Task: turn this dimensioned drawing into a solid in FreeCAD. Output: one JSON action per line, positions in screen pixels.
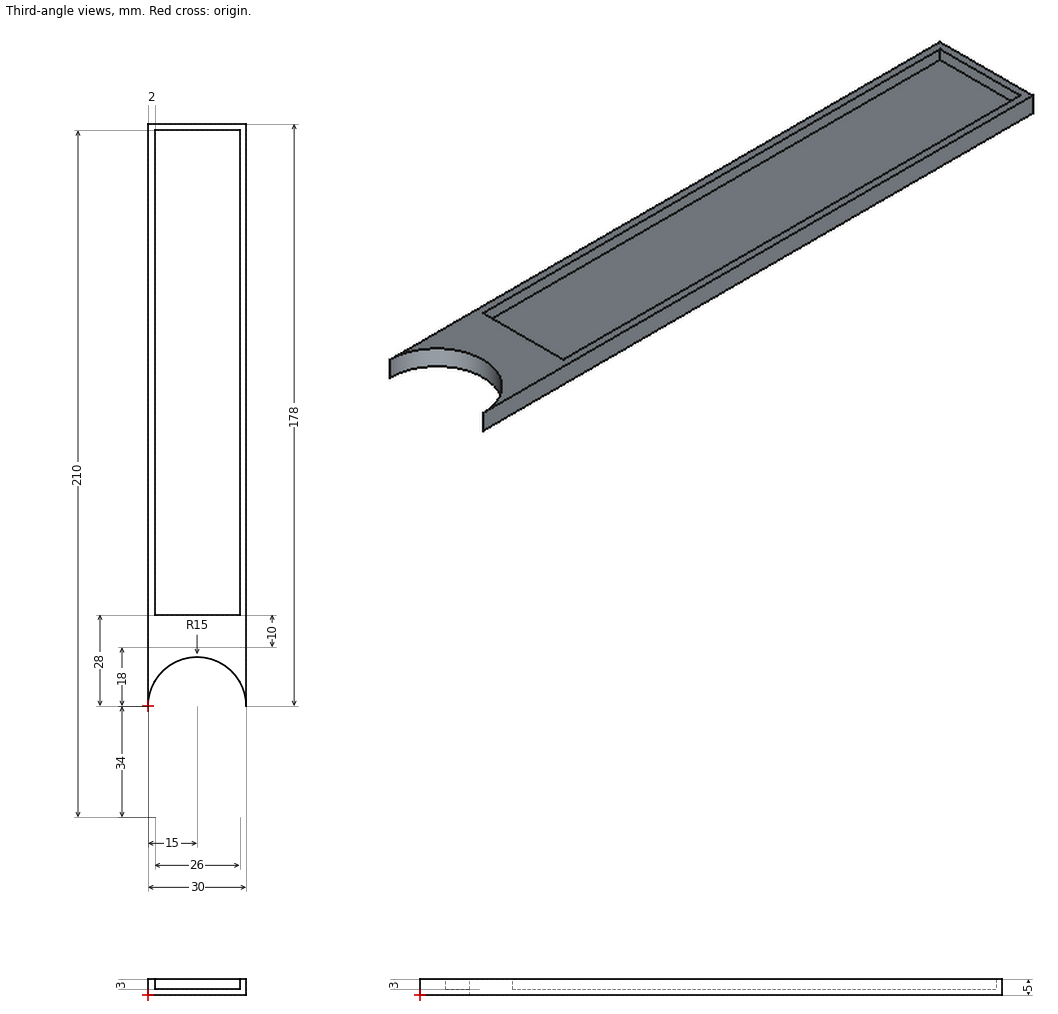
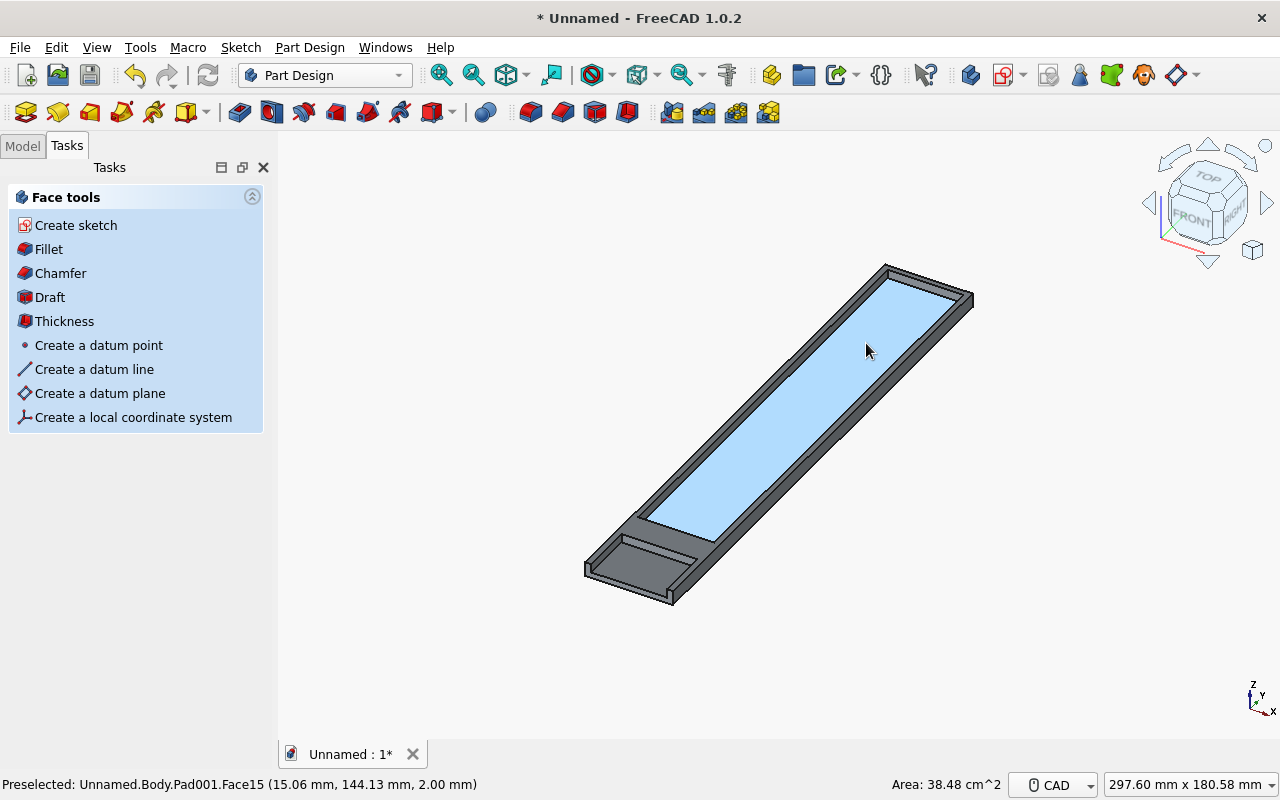
{"action": "left_click", "coordinate": [1004, 76]}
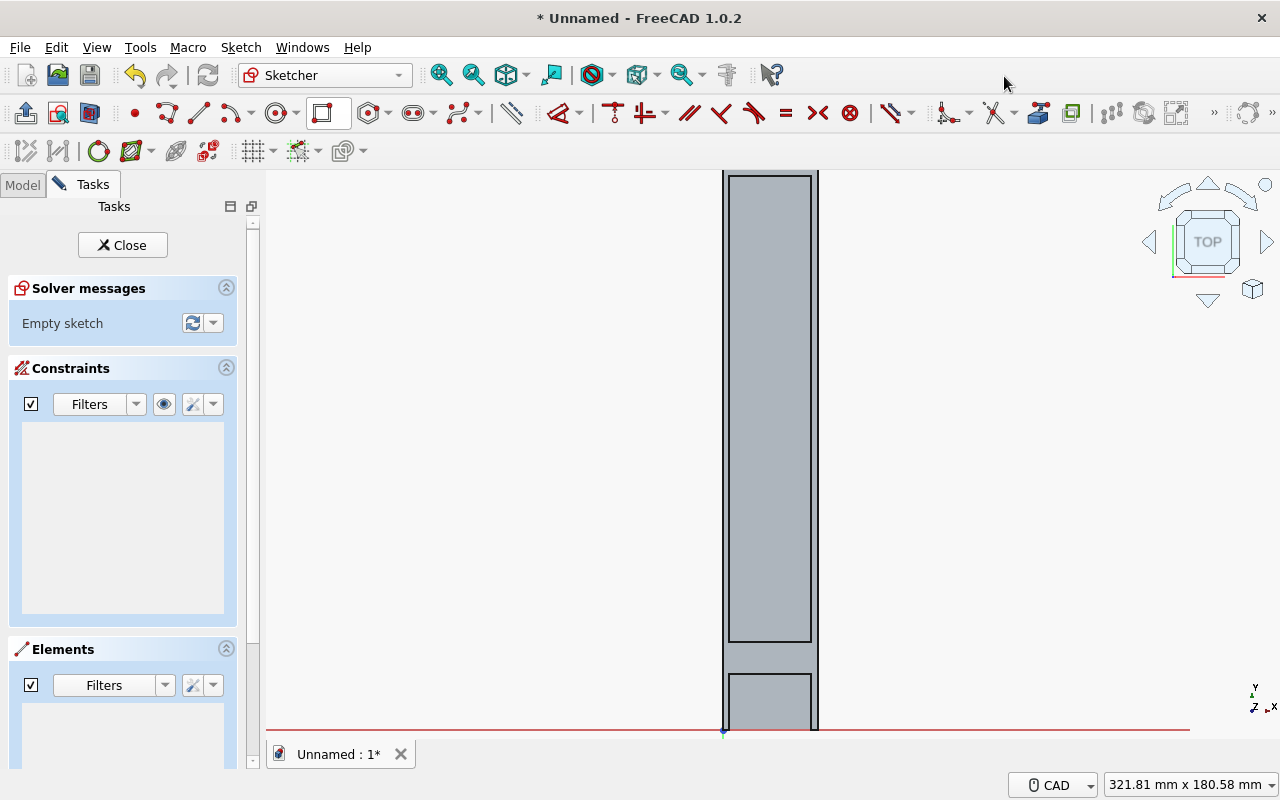
{"action": "scroll", "coordinate": [704, 454], "scroll_direction": "down", "scroll_amount": 5}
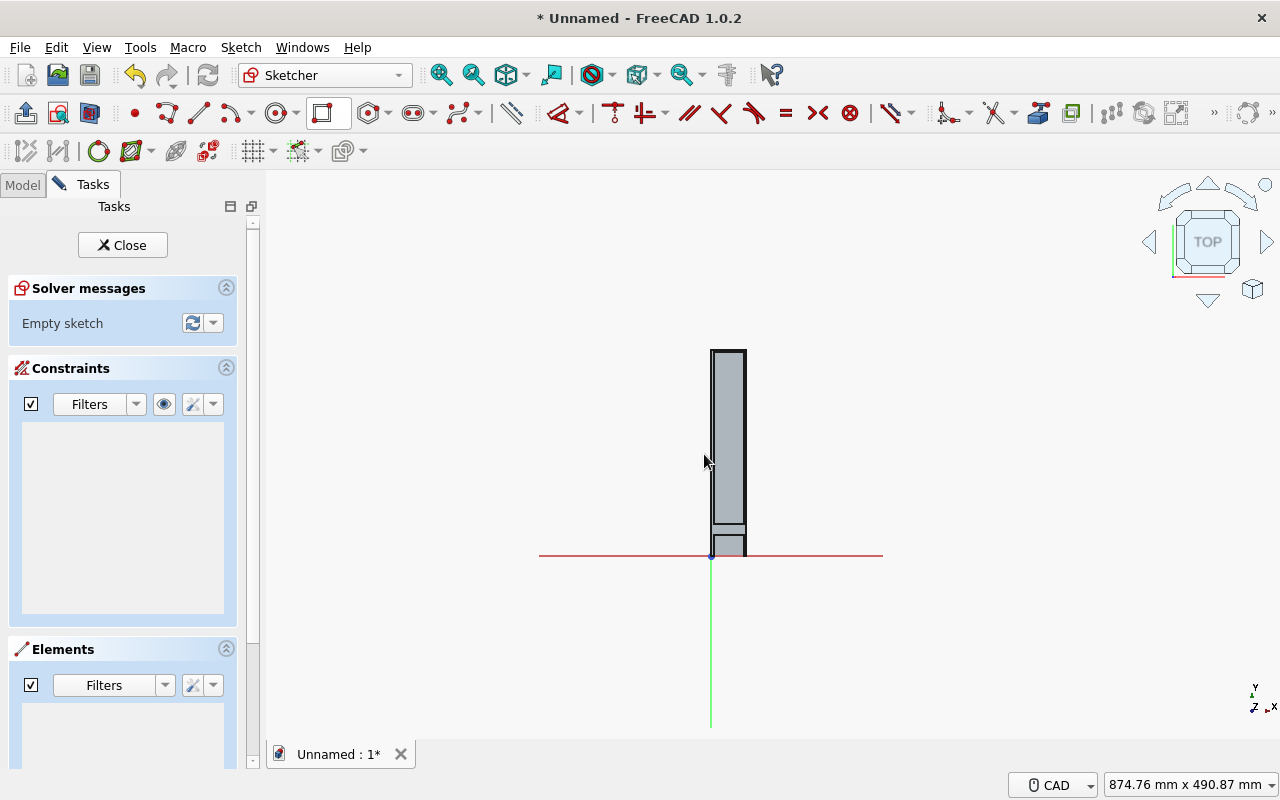
{"action": "scroll", "coordinate": [730, 553], "scroll_direction": "up", "scroll_amount": 14}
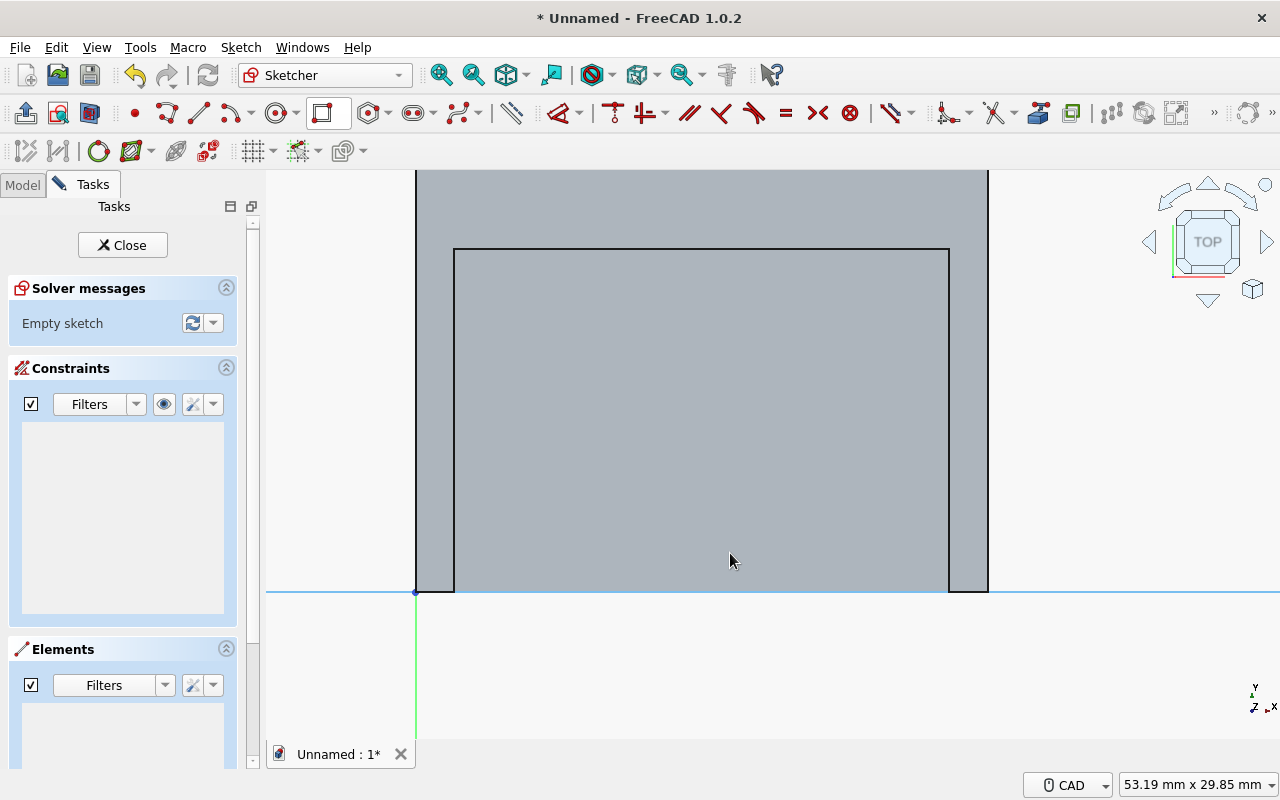
{"action": "key", "text": "g l"}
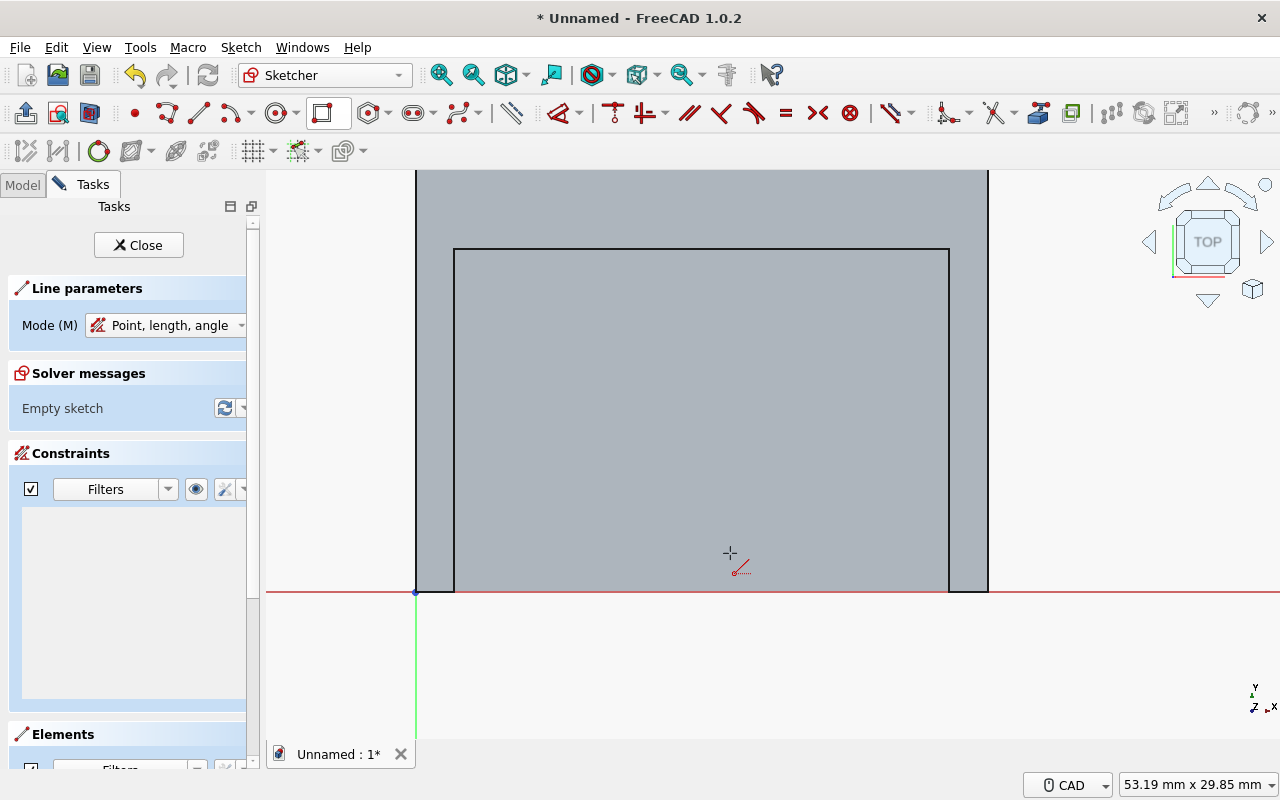
{"action": "left_click", "coordinate": [416, 592]}
{"action": "left_click", "coordinate": [988, 583]}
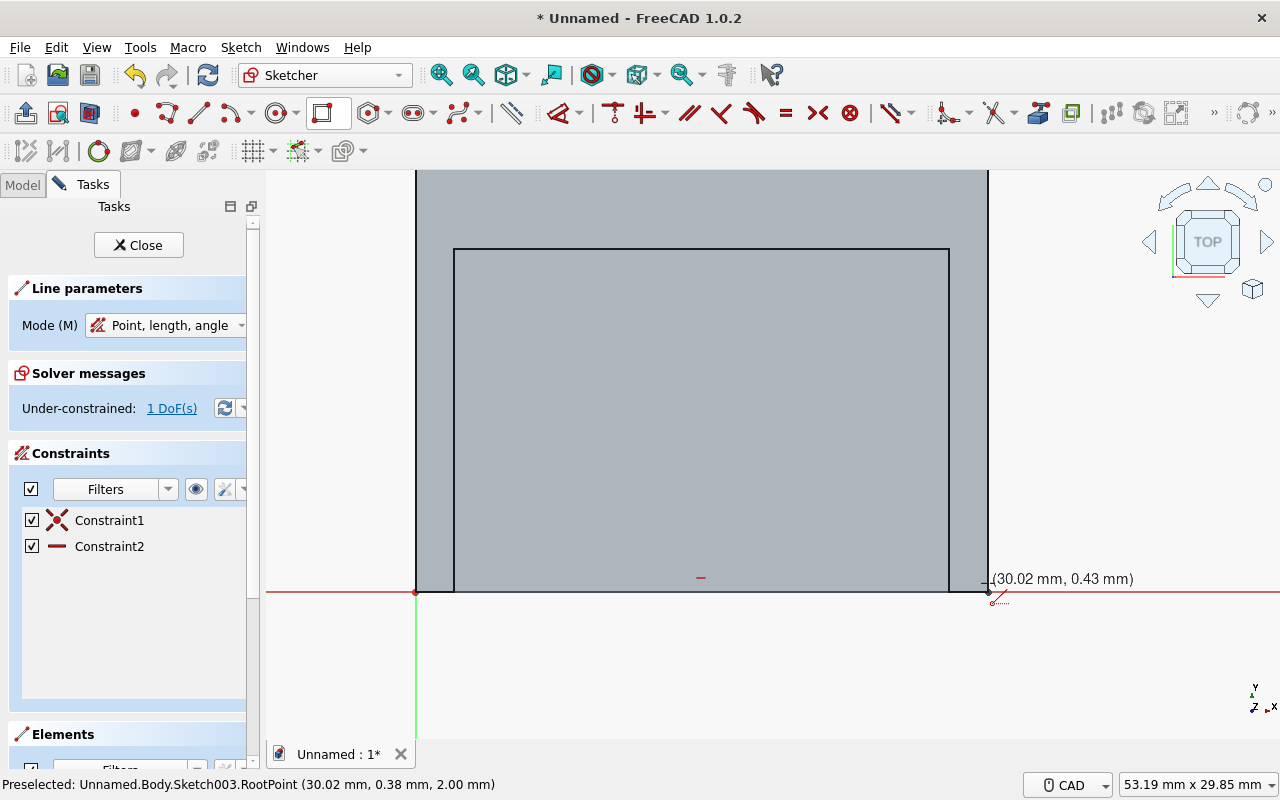
{"action": "key", "text": "g 3 a"}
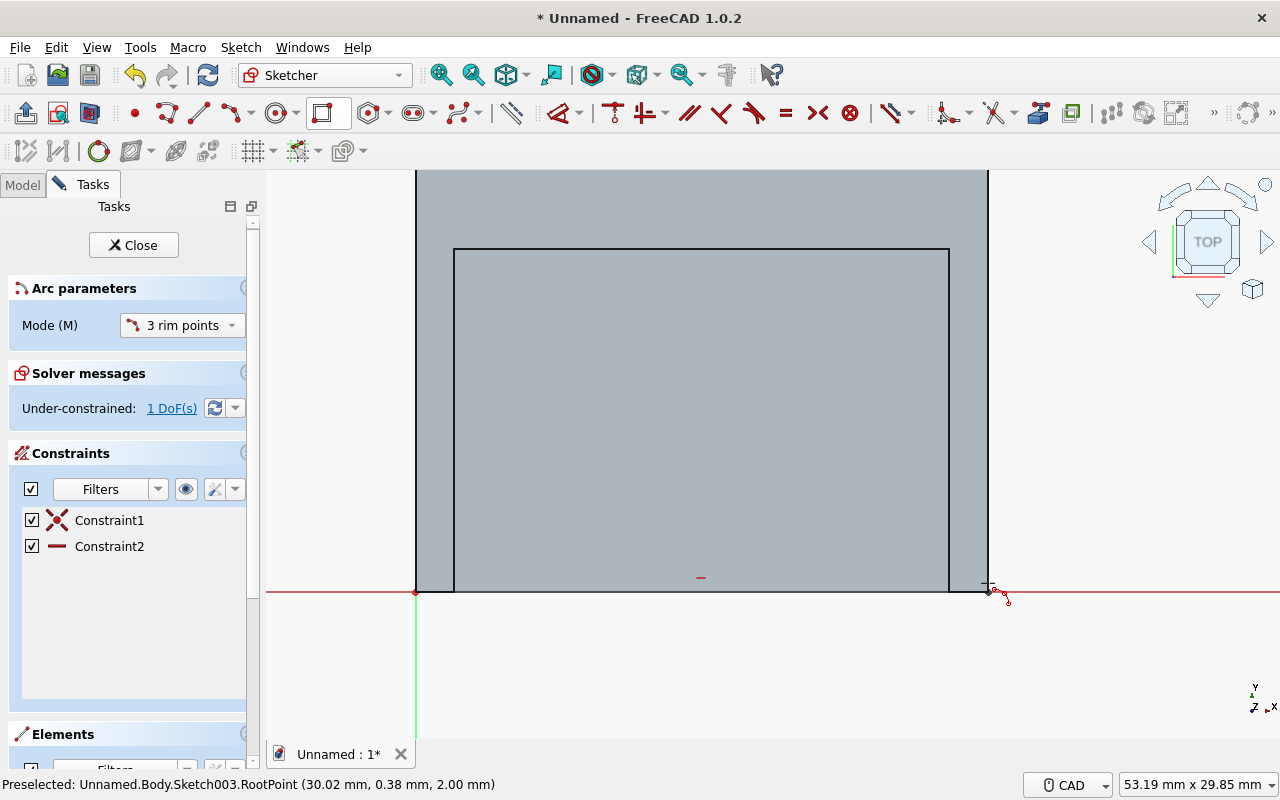
{"action": "left_click", "coordinate": [988, 583]}
{"action": "left_click", "coordinate": [416, 592]}
{"action": "left_click", "coordinate": [702, 306]}
{"action": "key", "text": "Escape"}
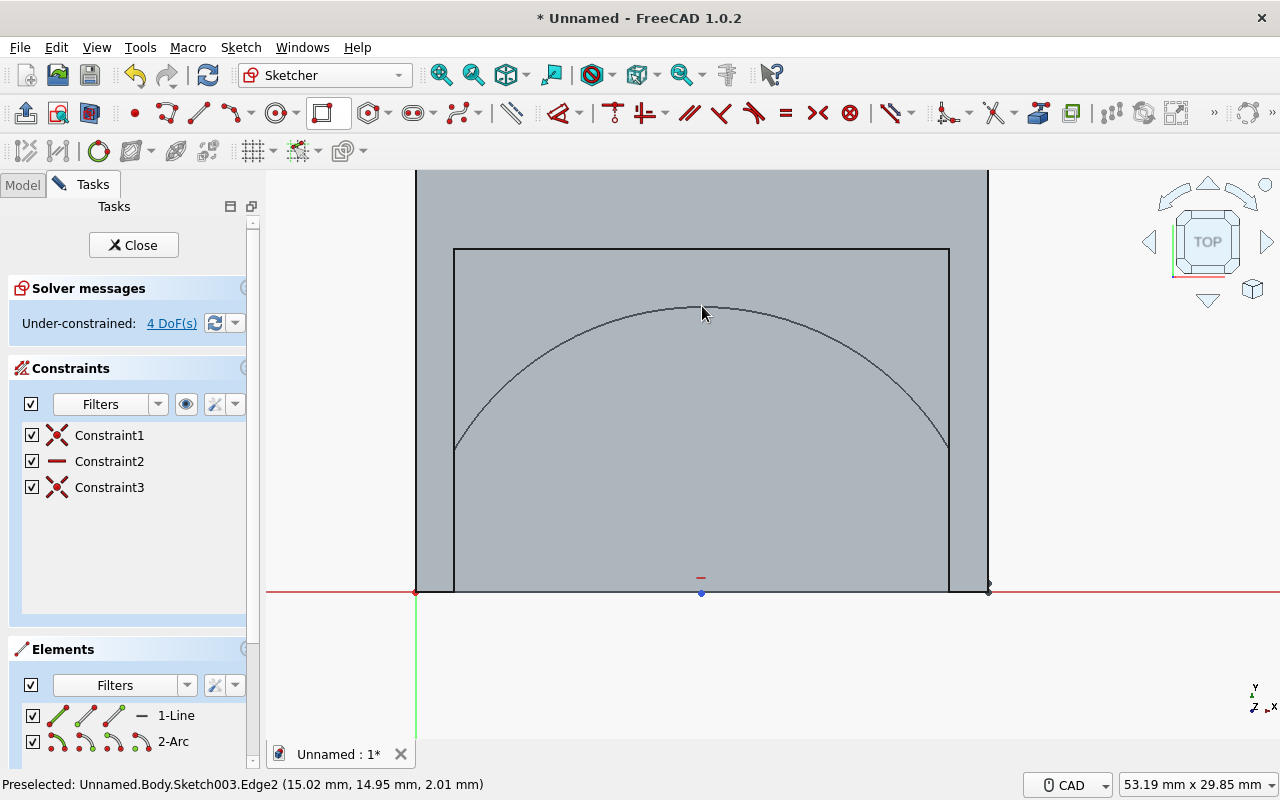
{"action": "left_click", "coordinate": [702, 593]}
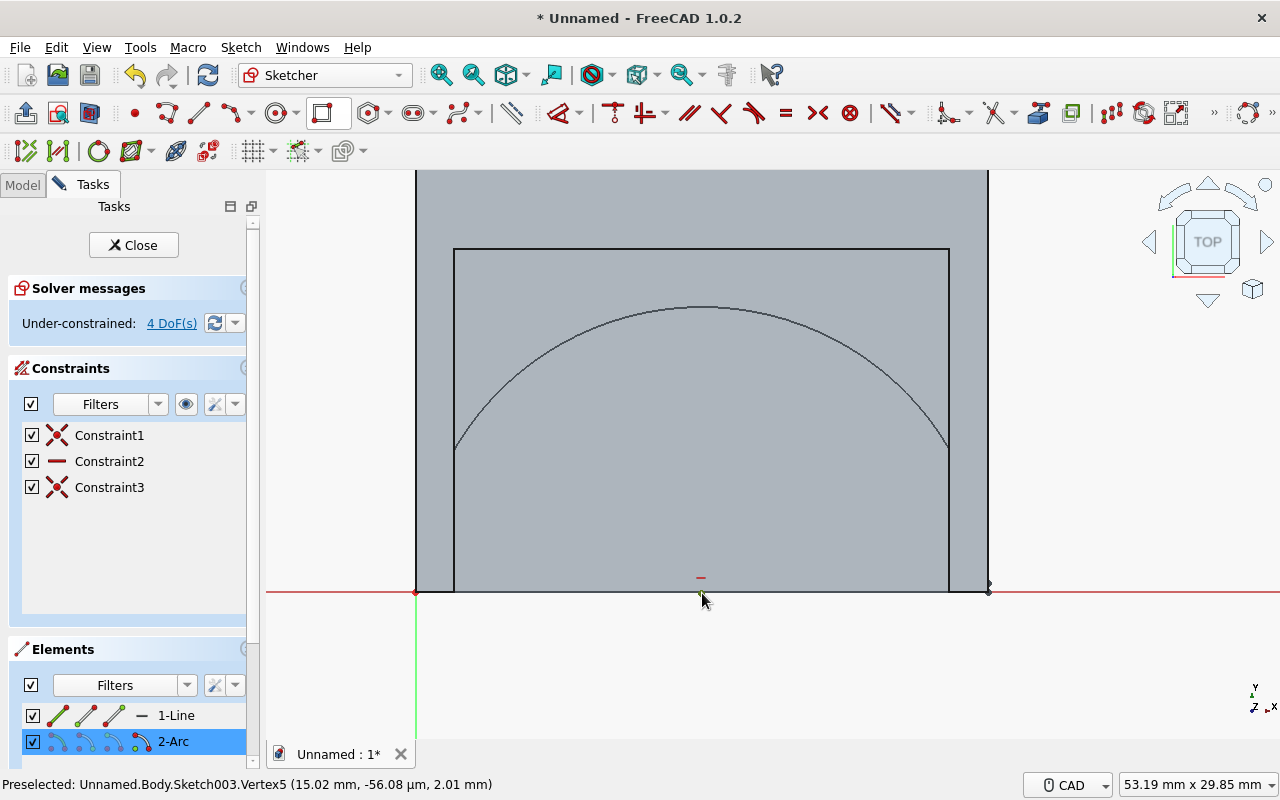
{"action": "left_click", "coordinate": [353, 592]}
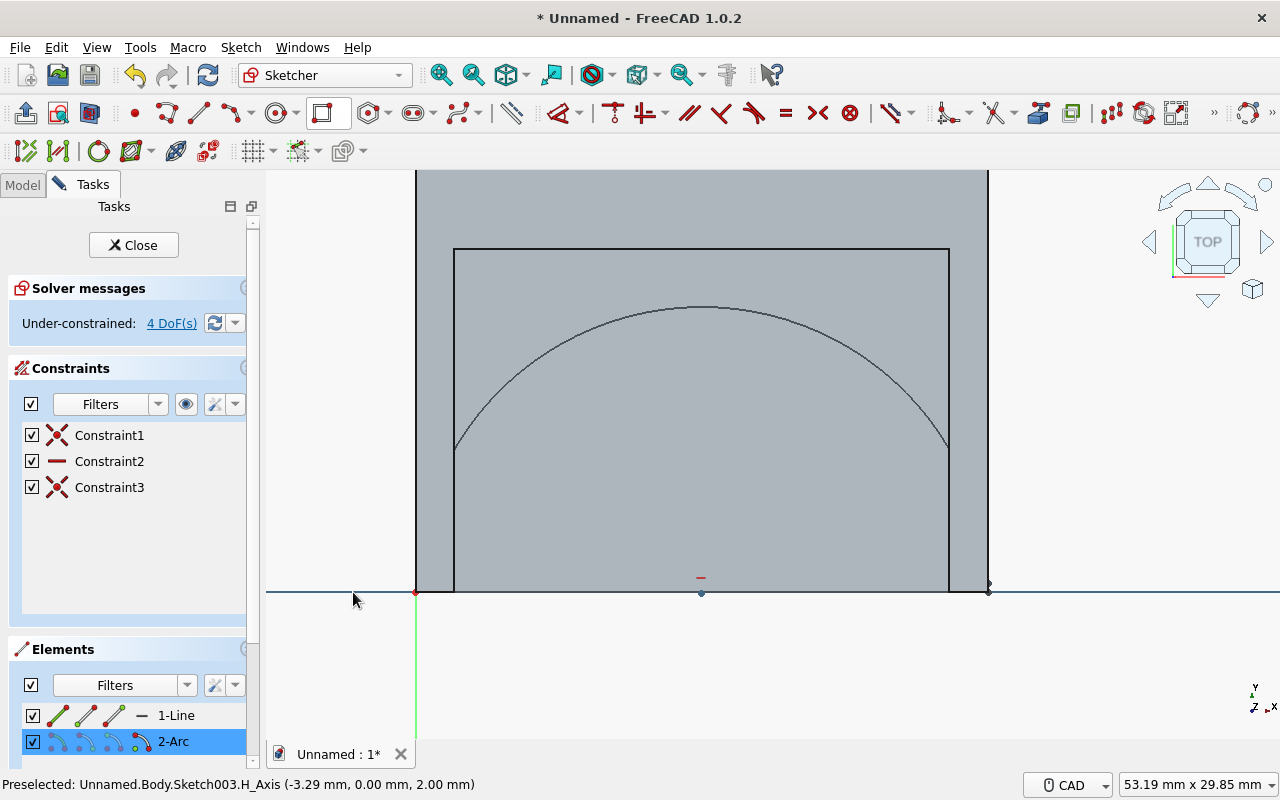
{"action": "key", "text": "c"}